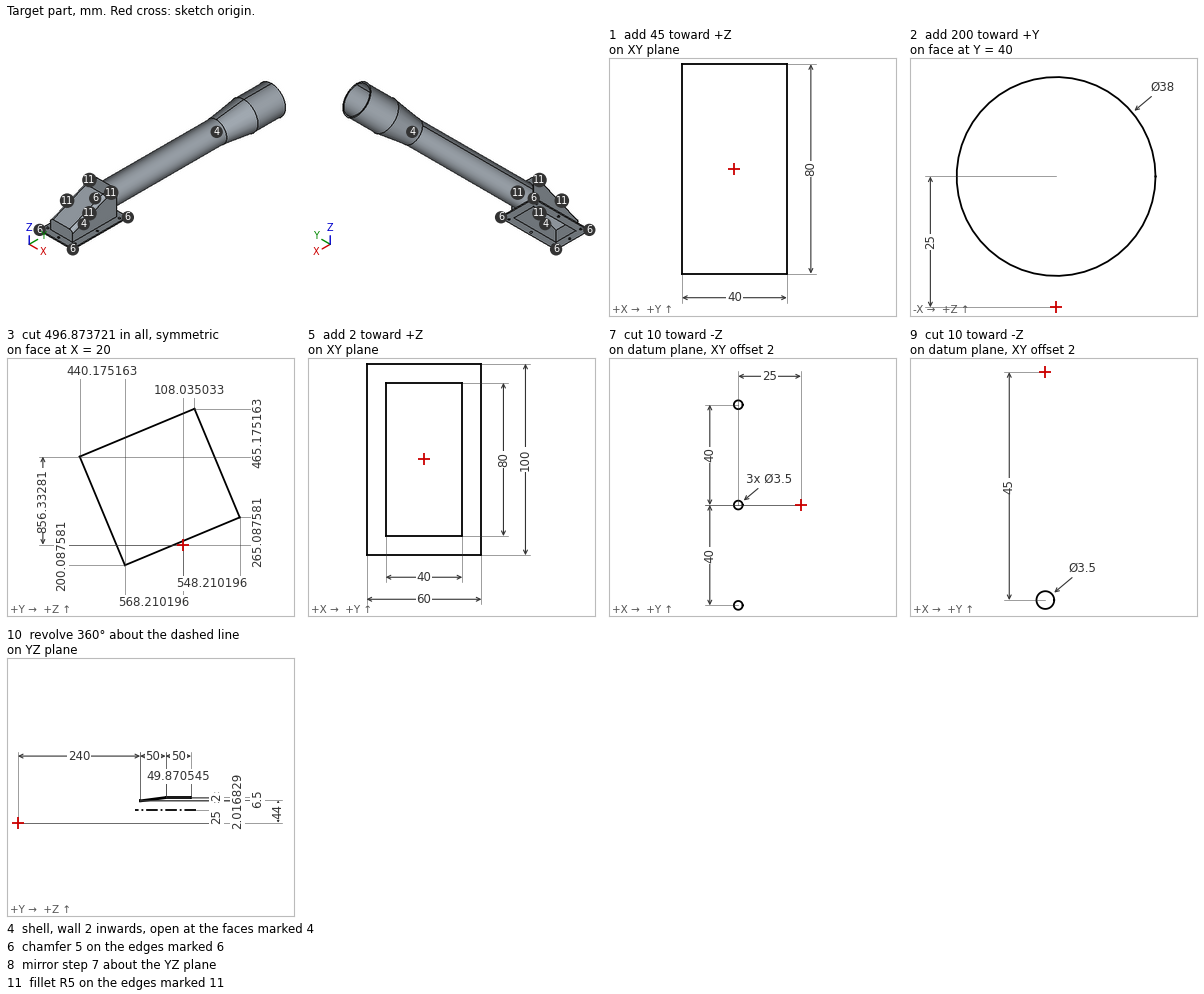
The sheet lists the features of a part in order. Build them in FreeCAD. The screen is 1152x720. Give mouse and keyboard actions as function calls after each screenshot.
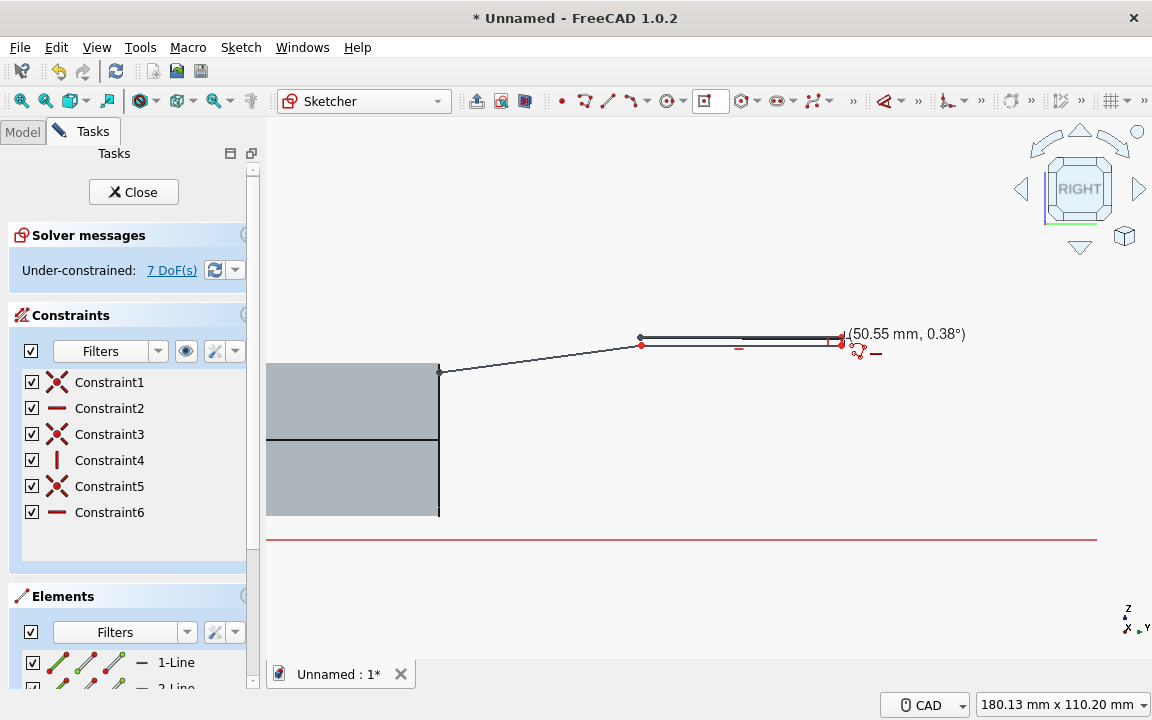
scroll(439, 363, up, 4)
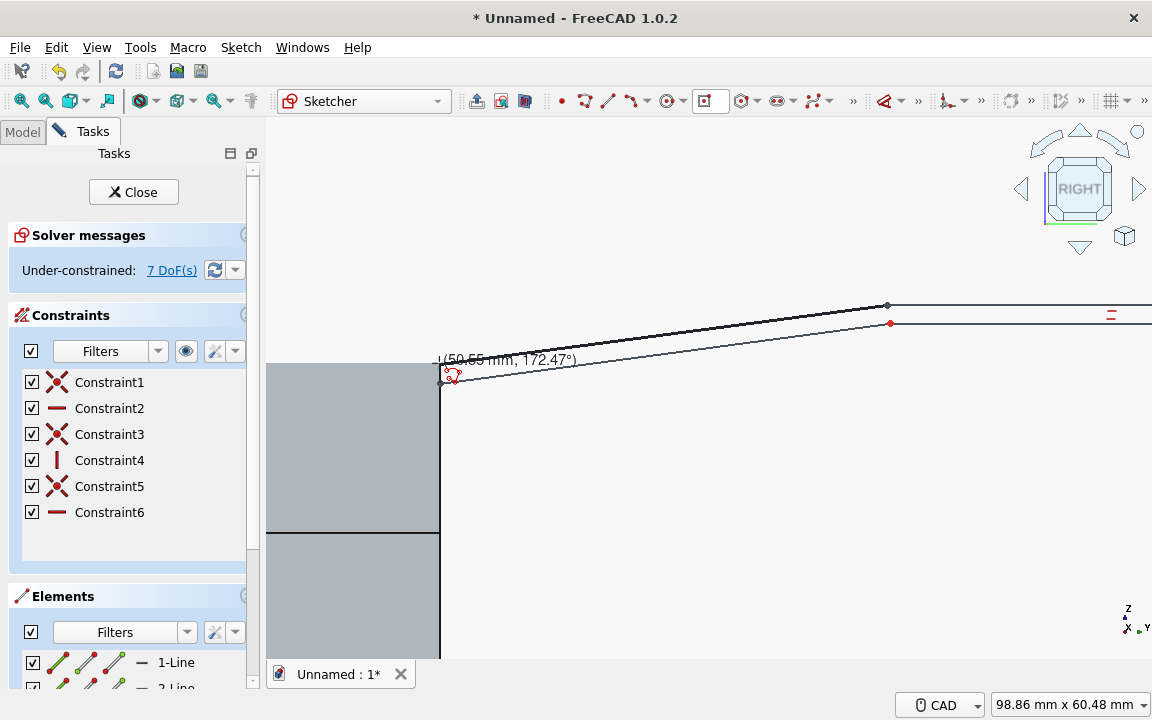
click(440, 363)
click(440, 384)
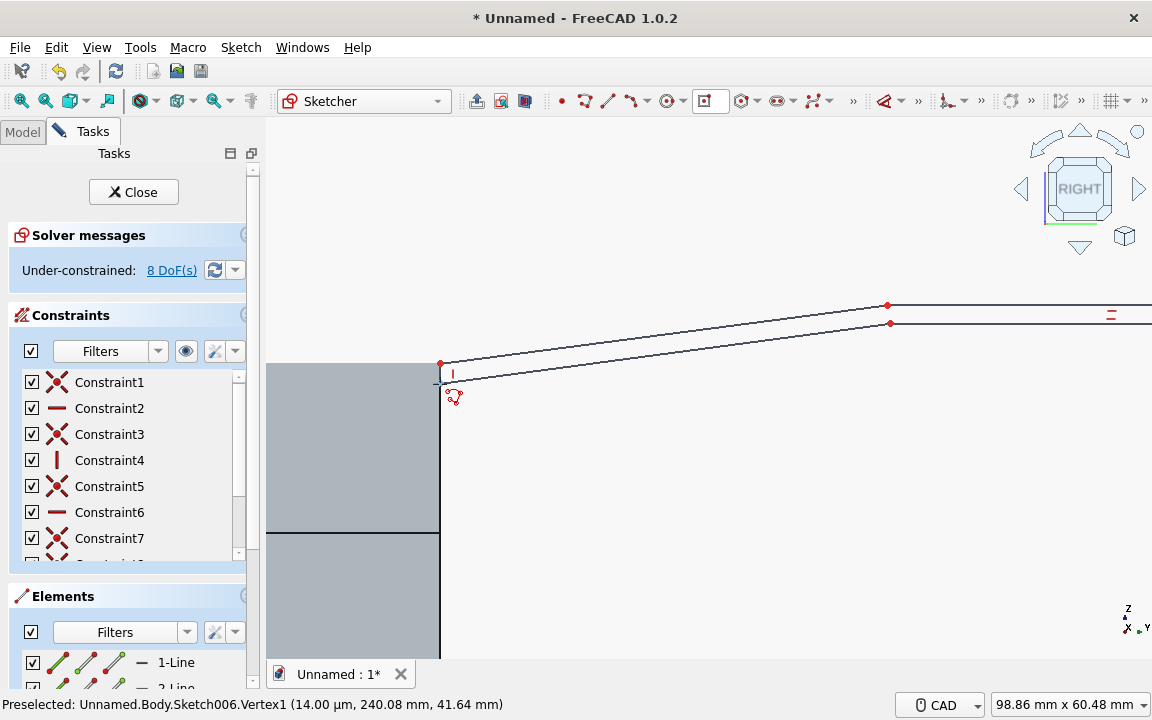
click(608, 102)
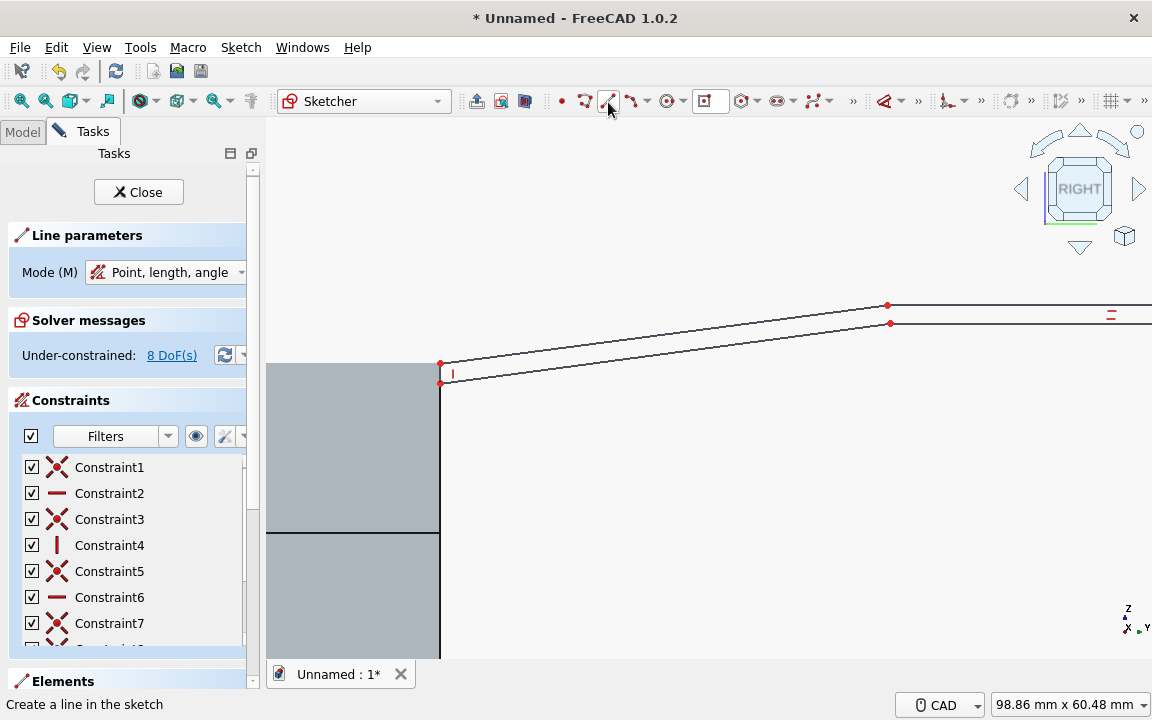
scroll(439, 363, down, 4)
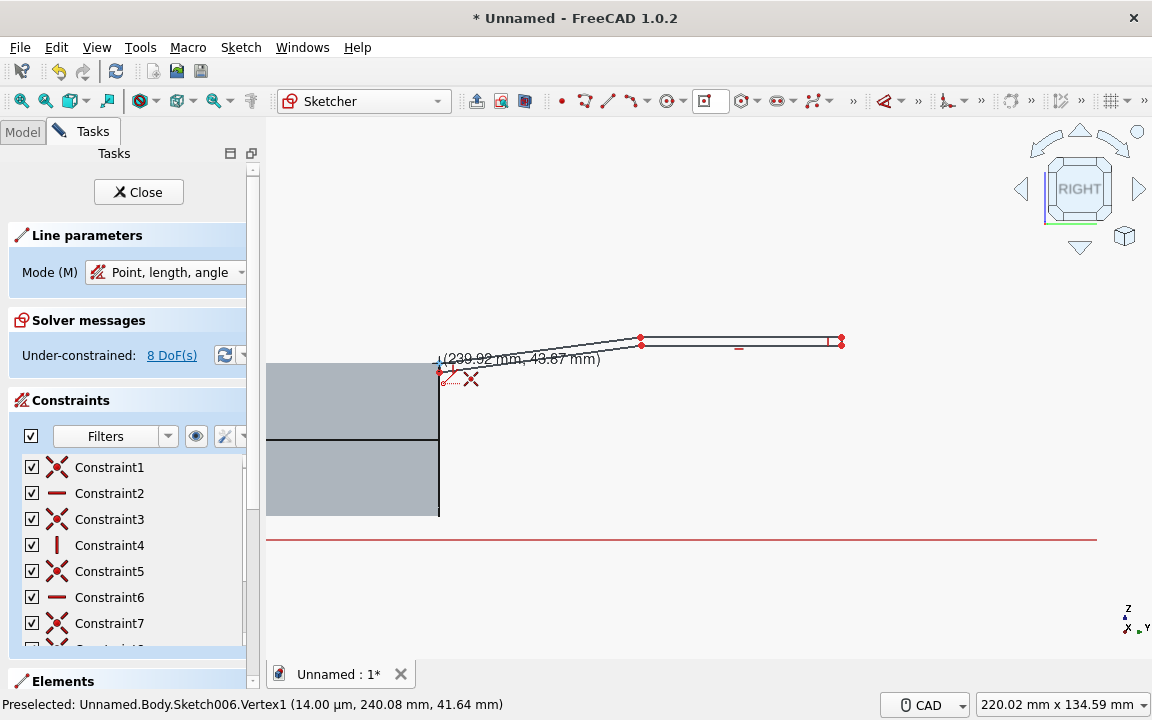
click(882, 440)
click(399, 440)
key(Escape)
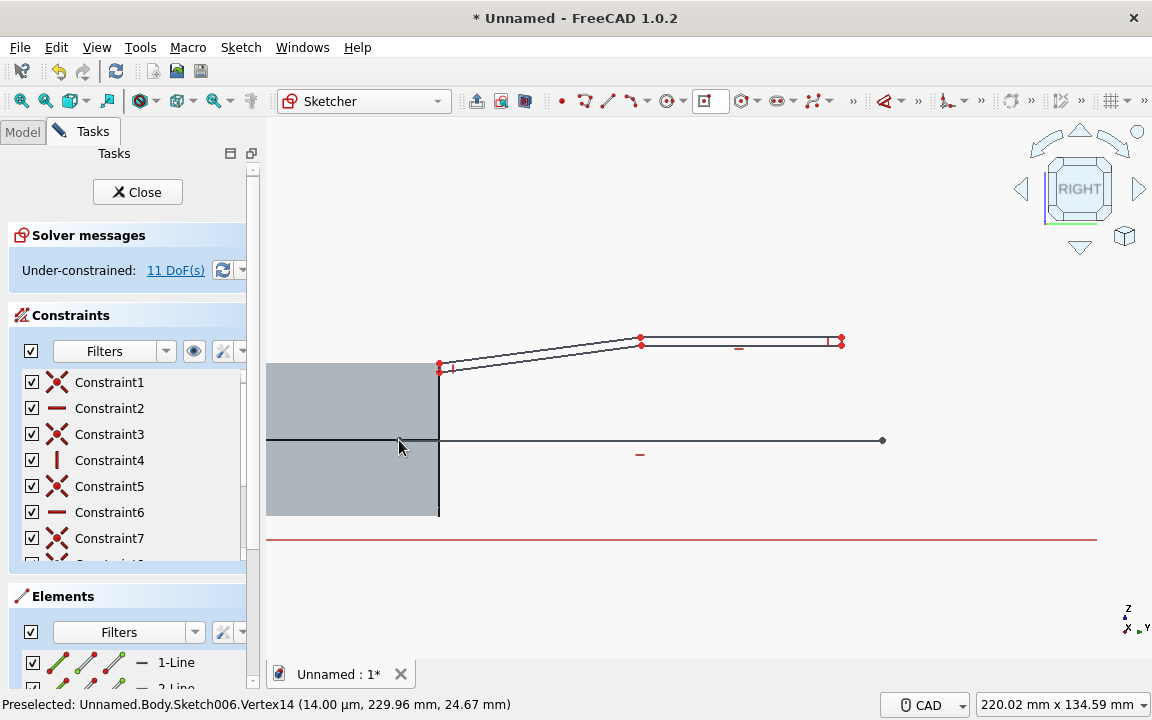
click(737, 441)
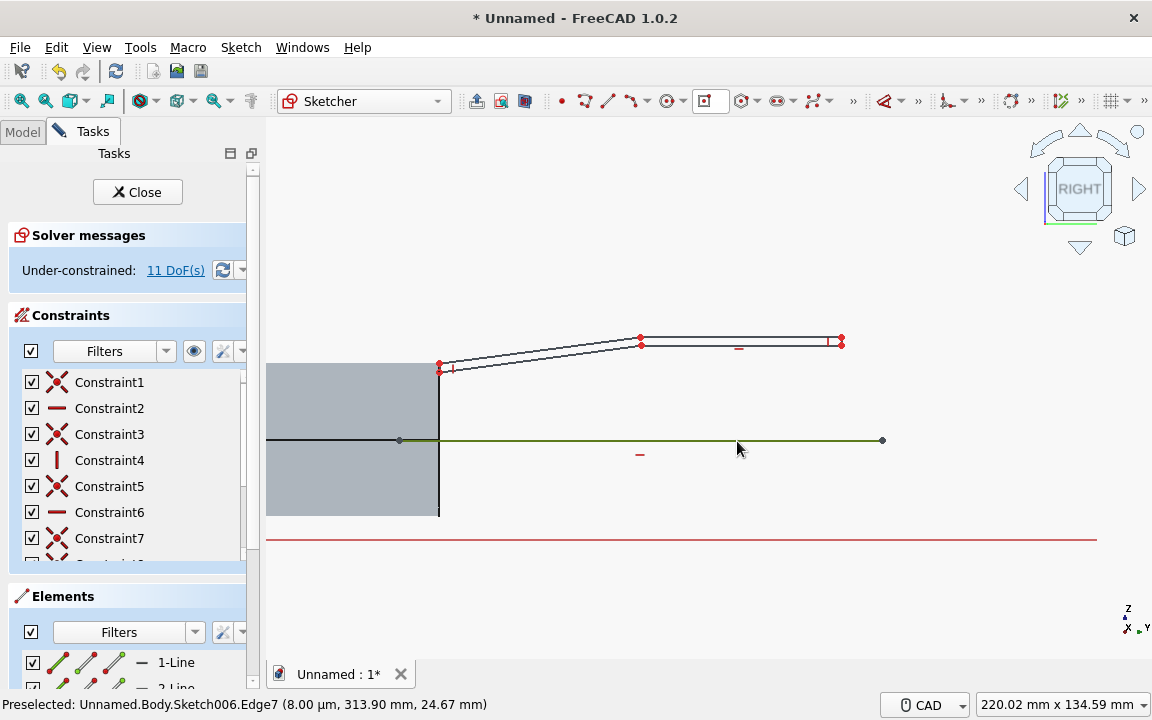
key(g)
key(n)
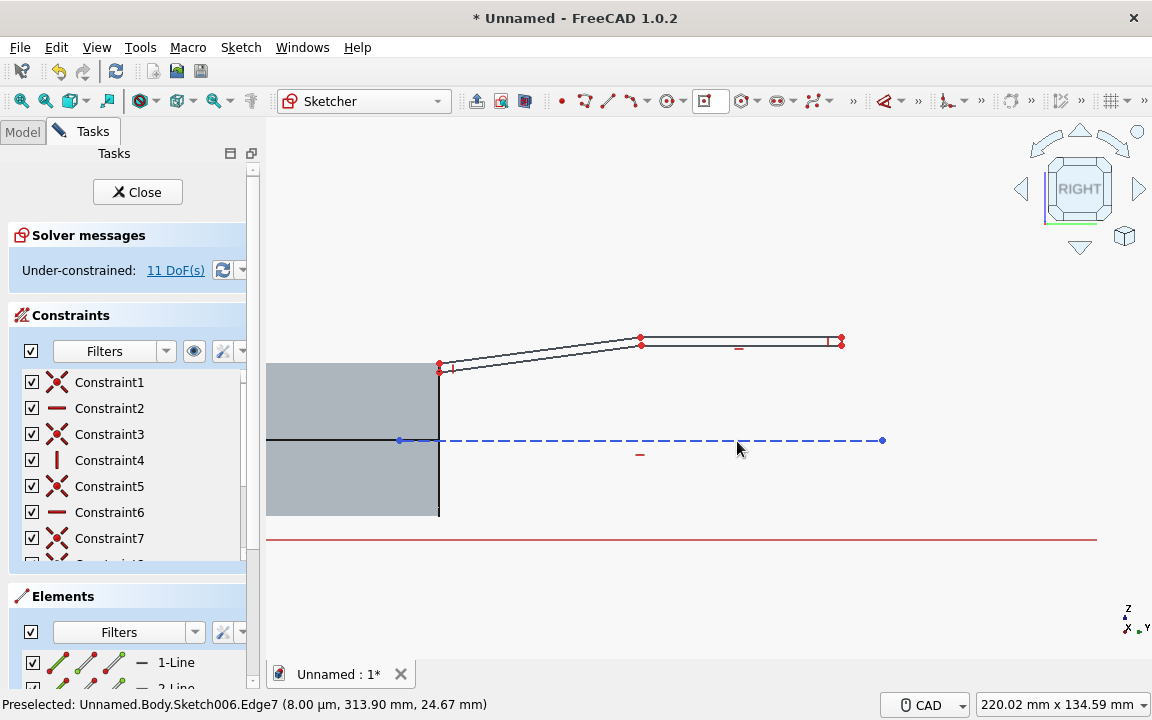
key(d)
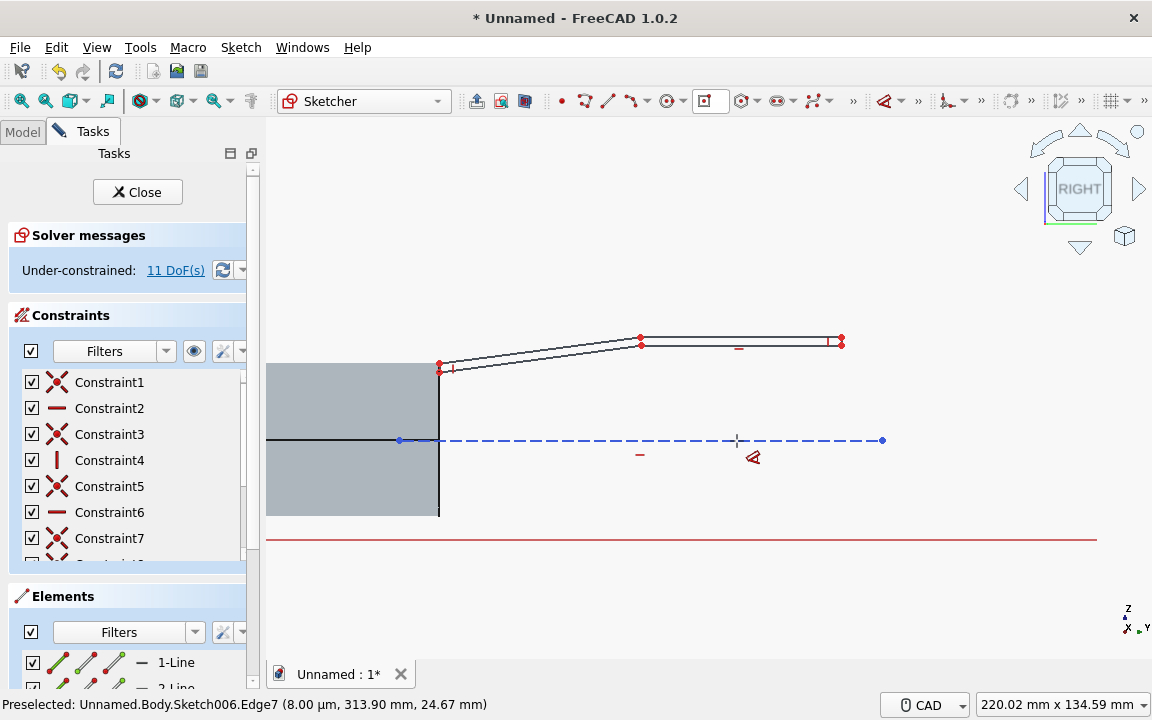
scroll(842, 341, up, 8)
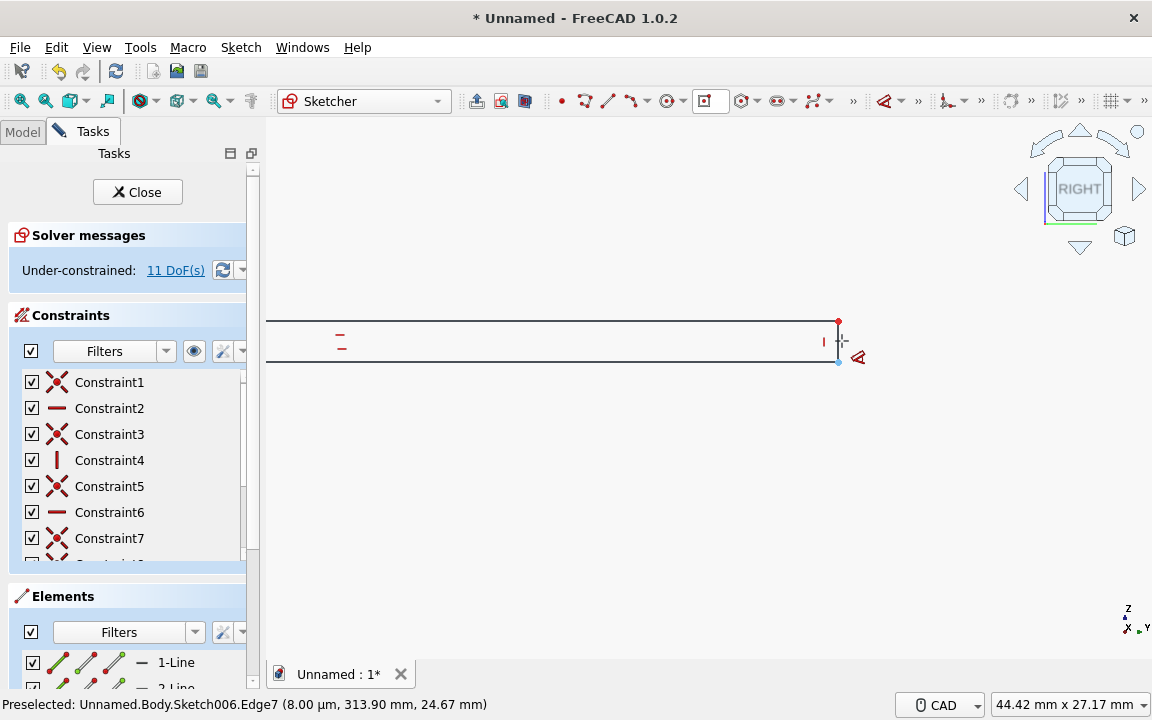
click(838, 342)
click(872, 342)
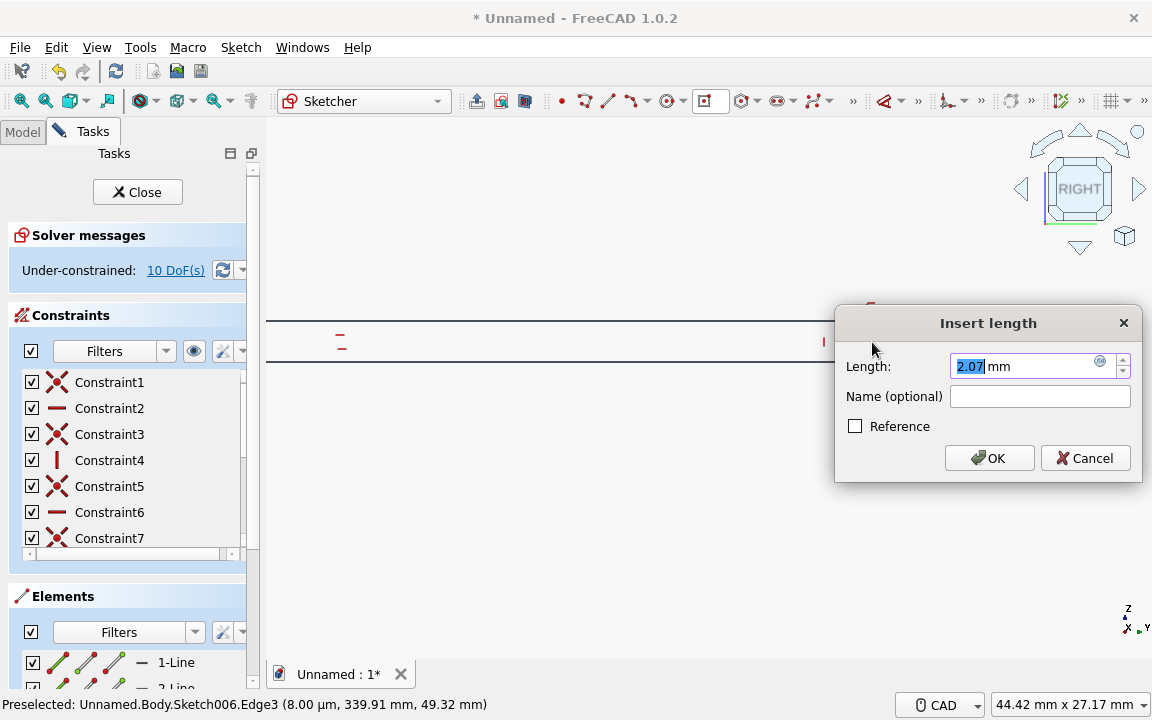
text(2)
key(Return)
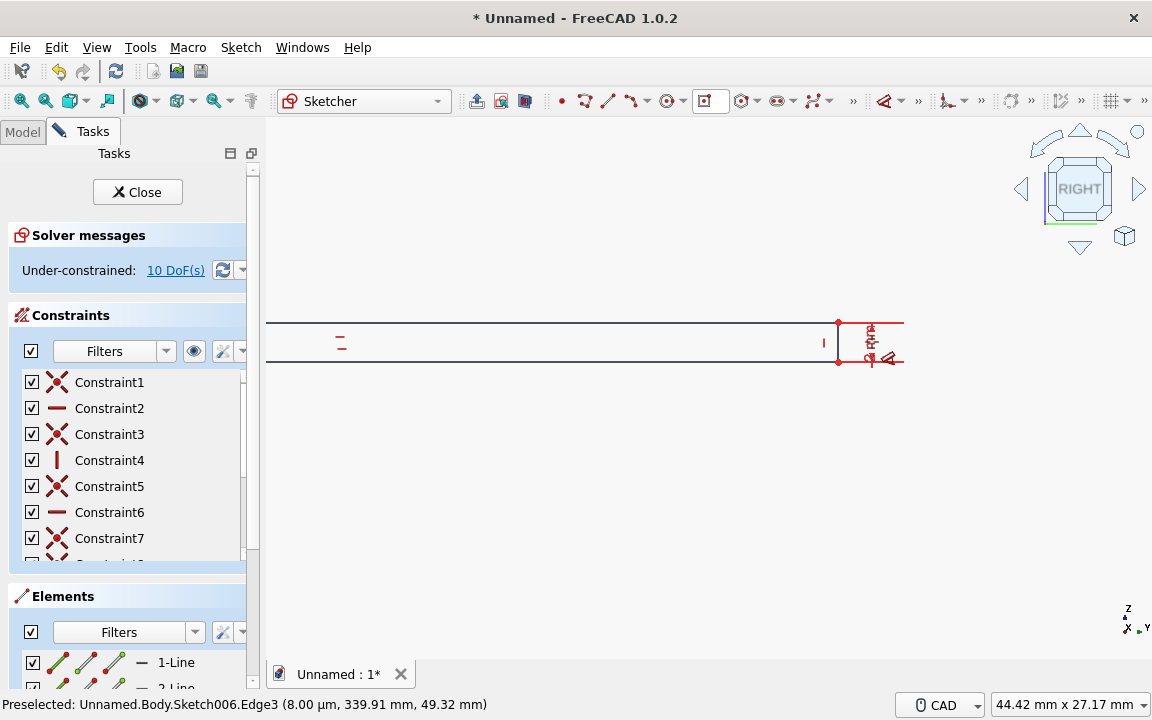
scroll(842, 341, down, 8)